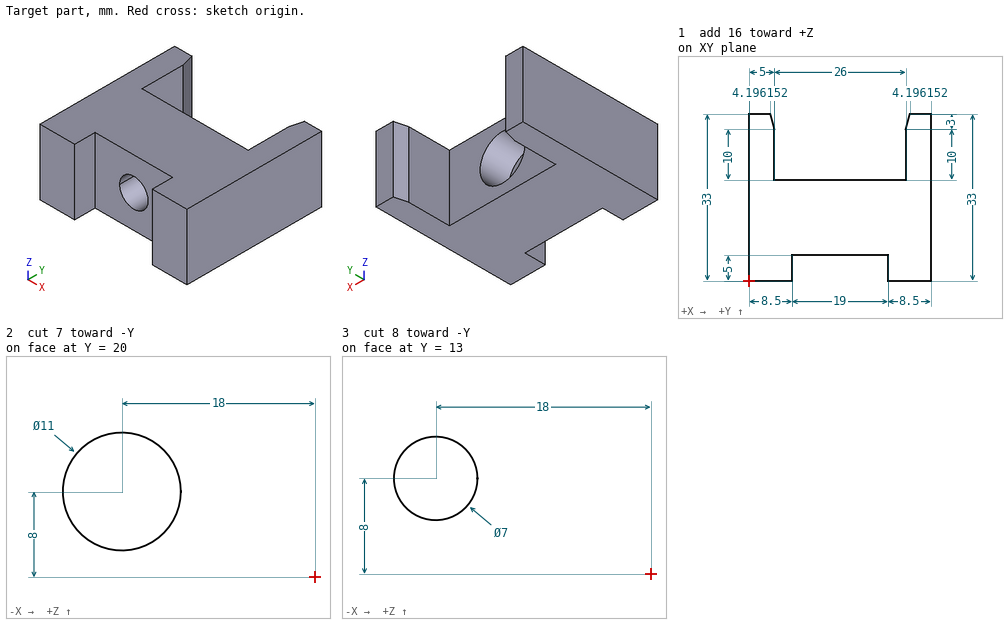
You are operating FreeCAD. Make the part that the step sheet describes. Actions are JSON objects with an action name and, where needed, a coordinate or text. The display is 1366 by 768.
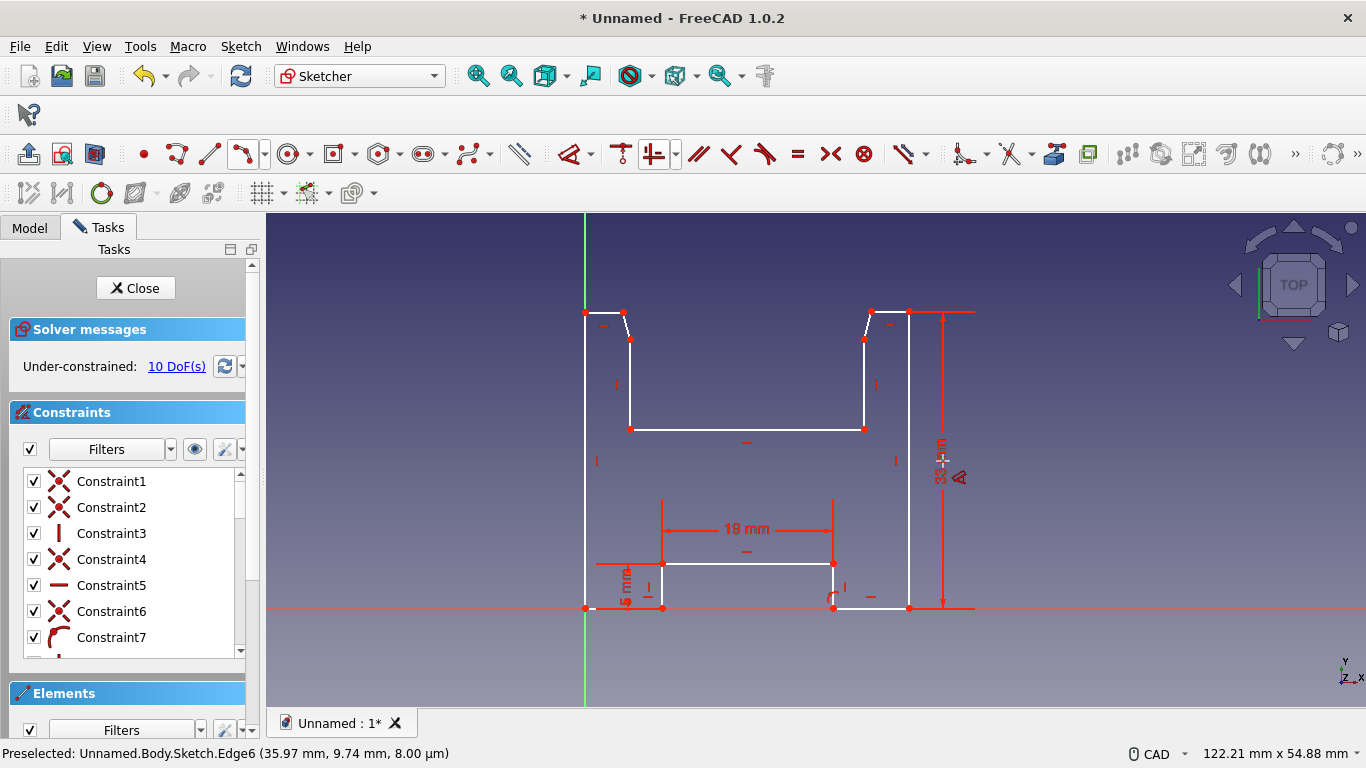
{"action": "left_click", "coordinate": [864, 367]}
{"action": "left_click", "coordinate": [830, 385]}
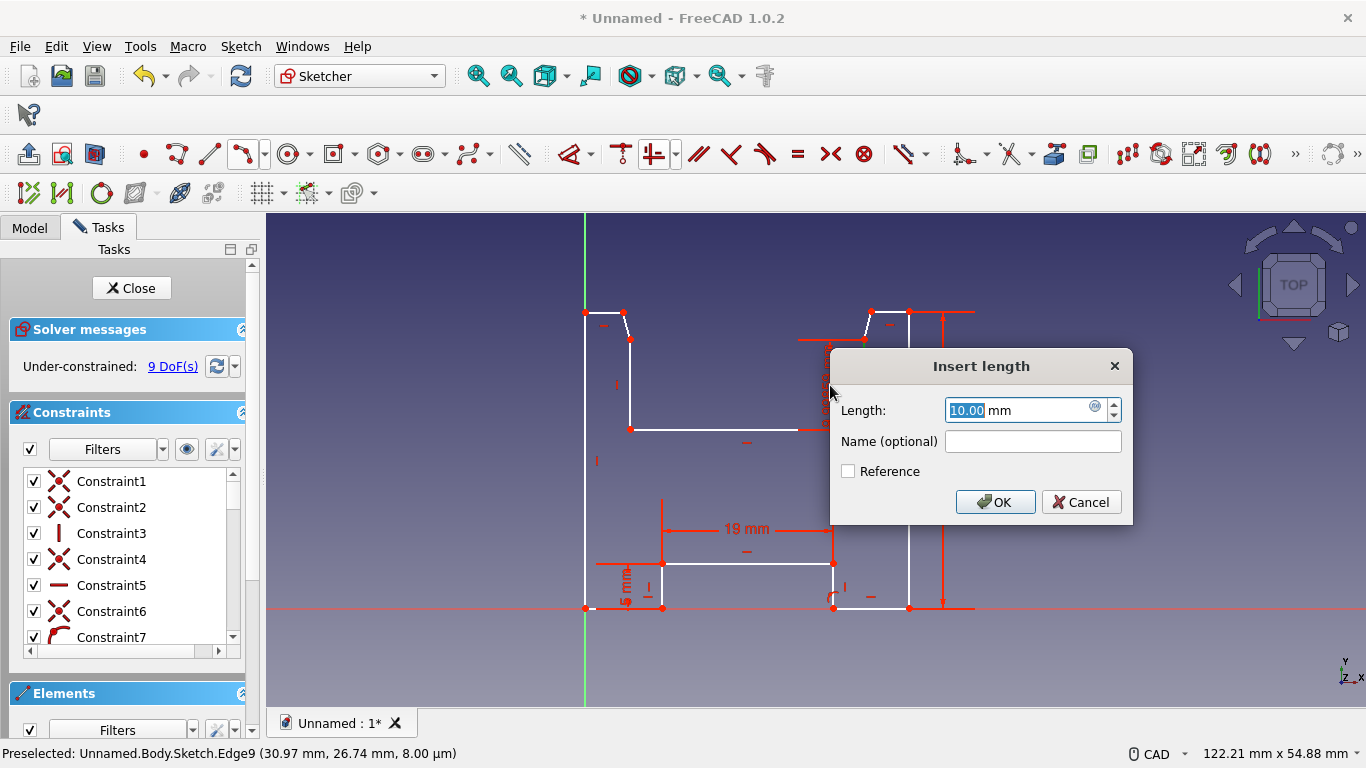
{"action": "type", "text": "10"}
{"action": "key", "text": "Return"}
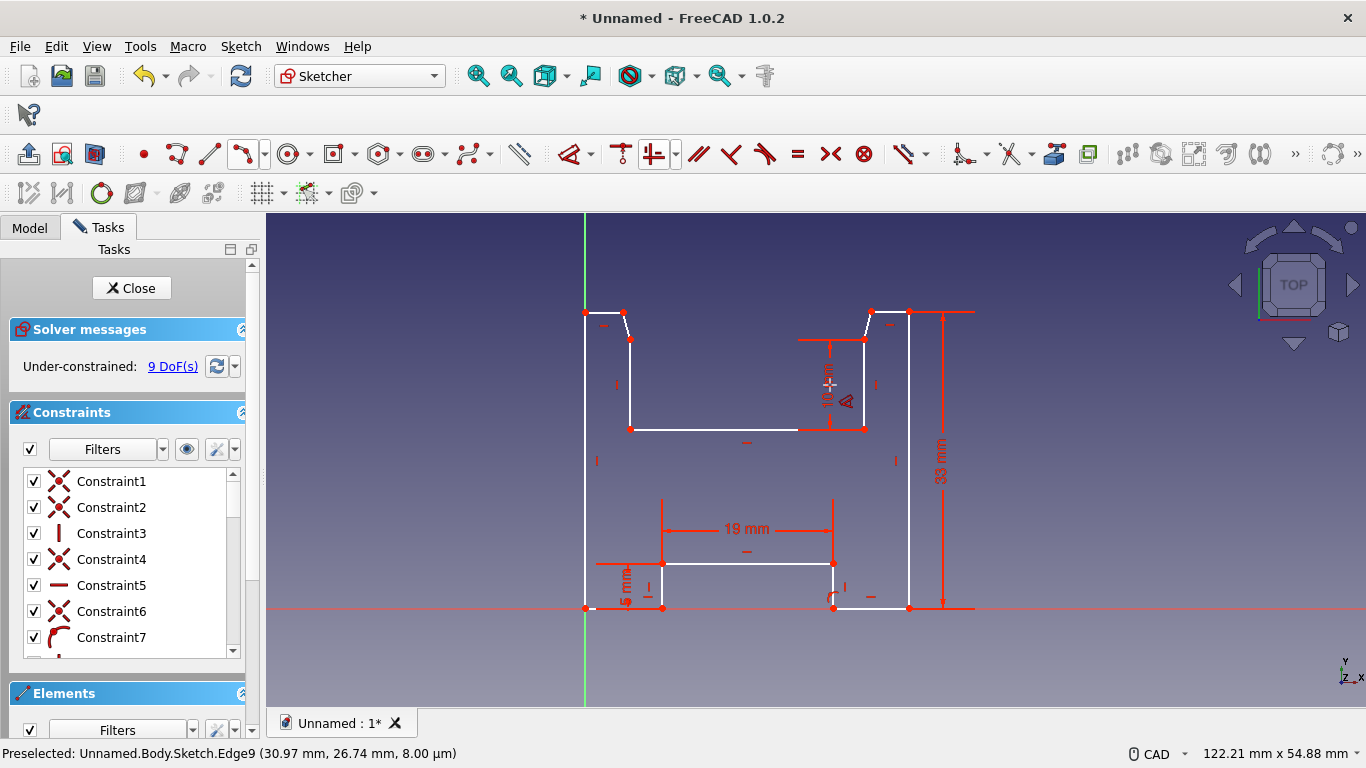
{"action": "left_click", "coordinate": [794, 430]}
{"action": "left_click", "coordinate": [747, 396]}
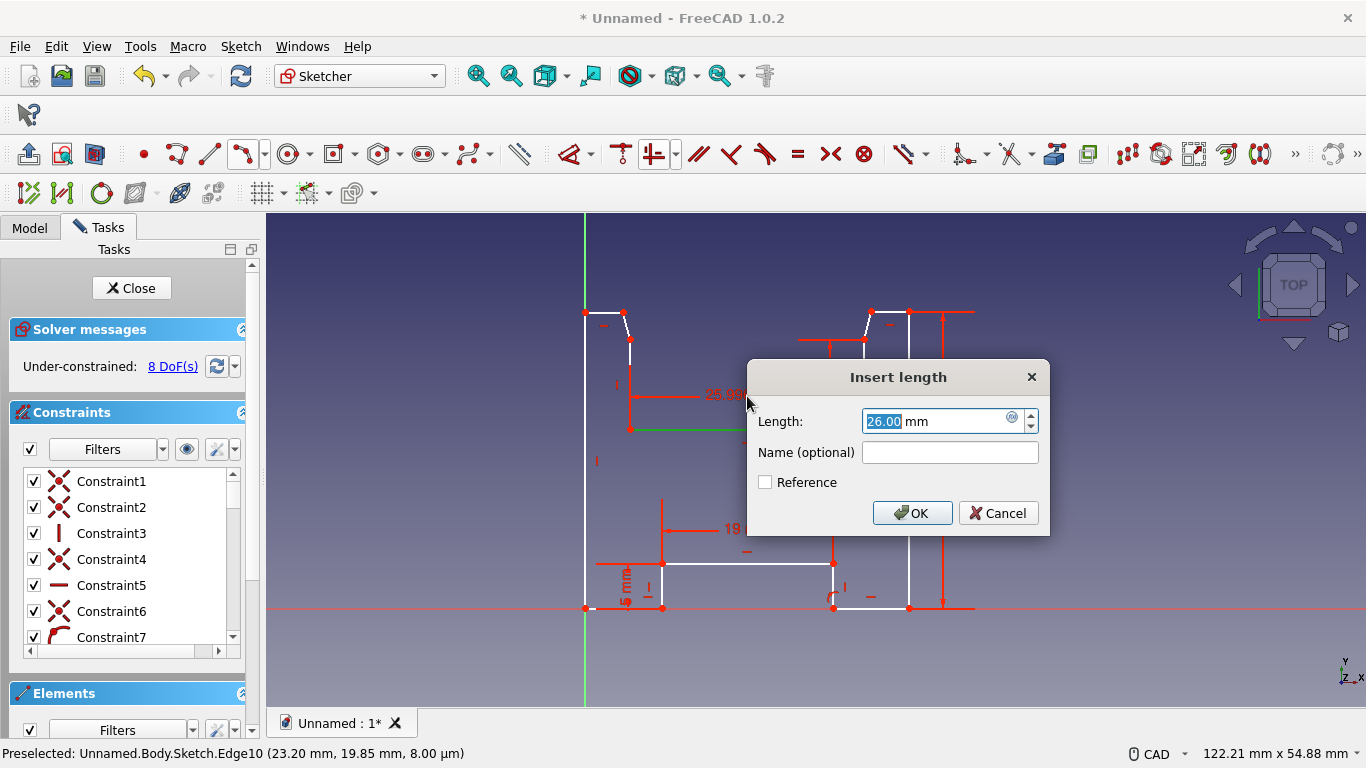
{"action": "type", "text": "26"}
{"action": "key", "text": "Return"}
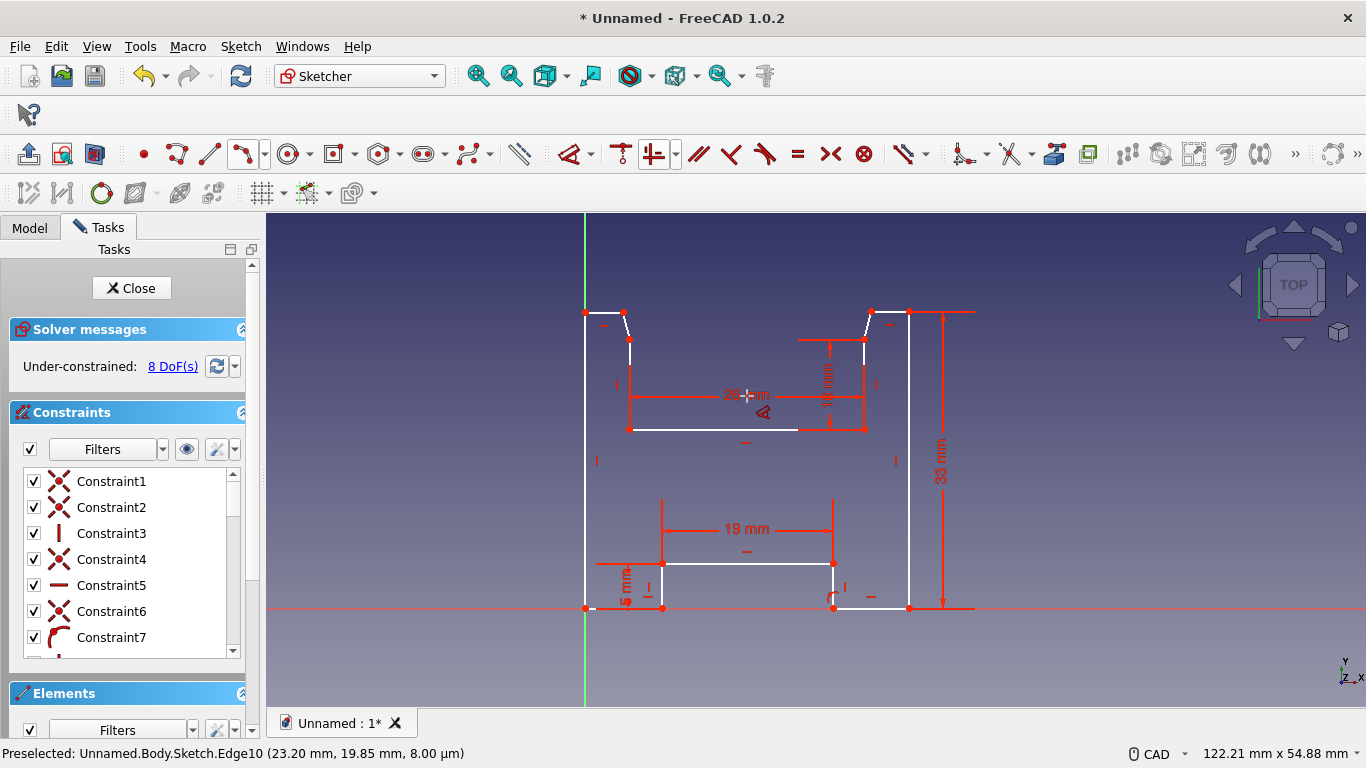
{"action": "left_click", "coordinate": [630, 403]}
{"action": "left_click", "coordinate": [664, 385]}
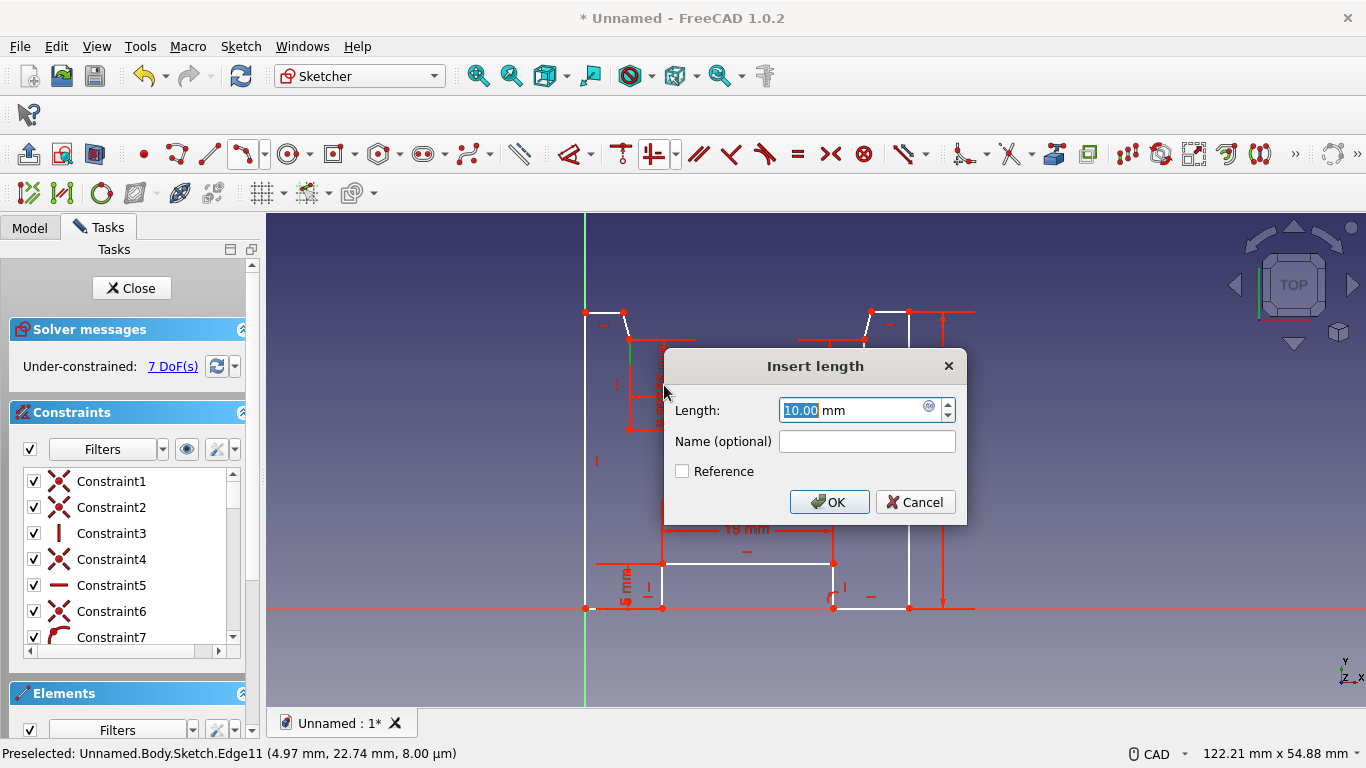
{"action": "type", "text": "10"}
{"action": "key", "text": "Return"}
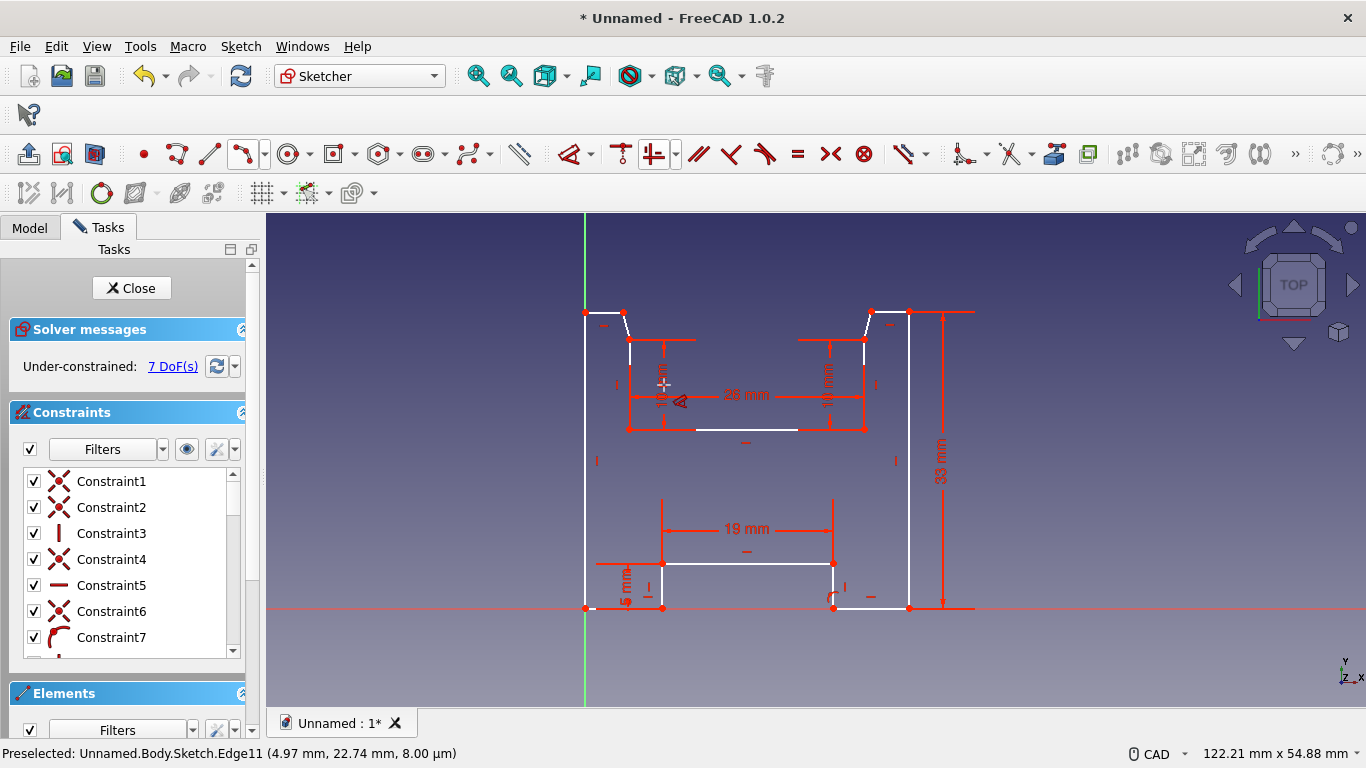
{"action": "left_click", "coordinate": [585, 402]}
{"action": "left_click", "coordinate": [551, 461]}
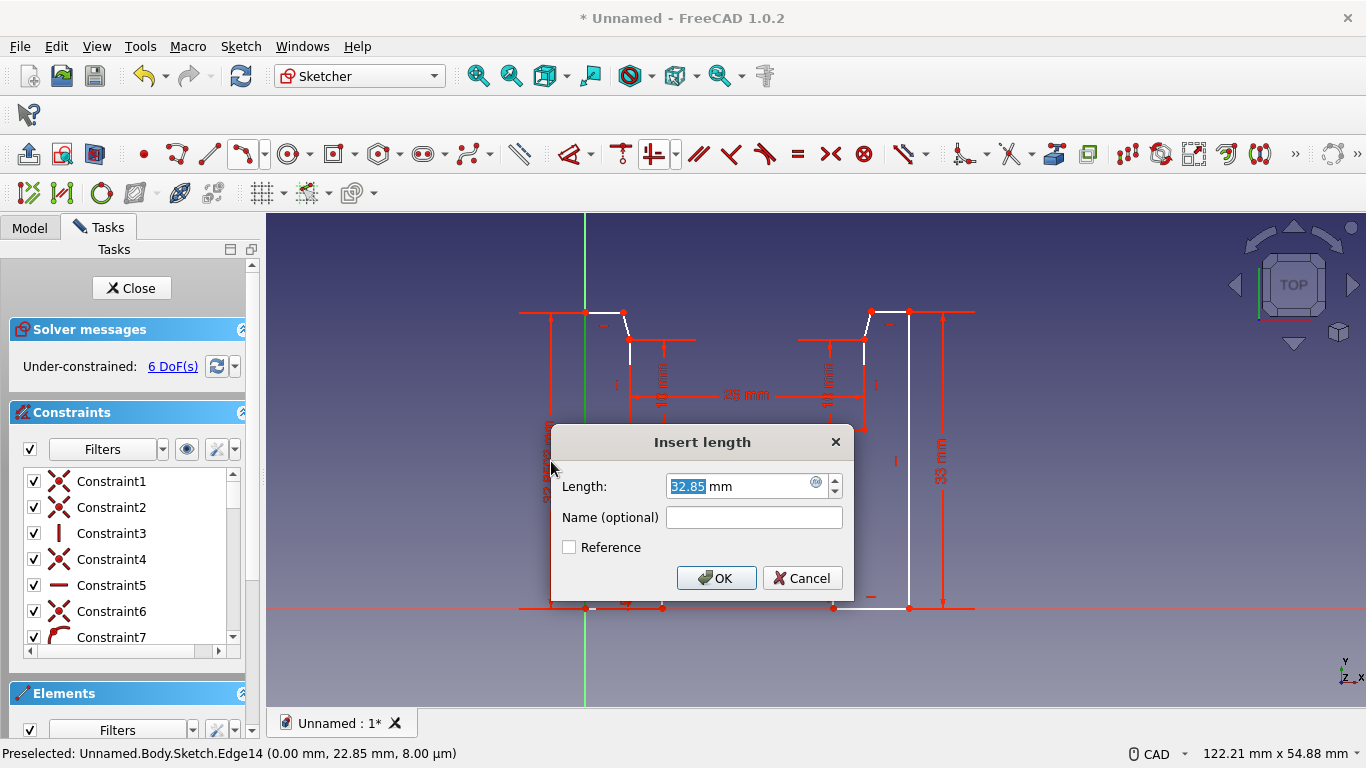
{"action": "type", "text": "33"}
{"action": "key", "text": "Return"}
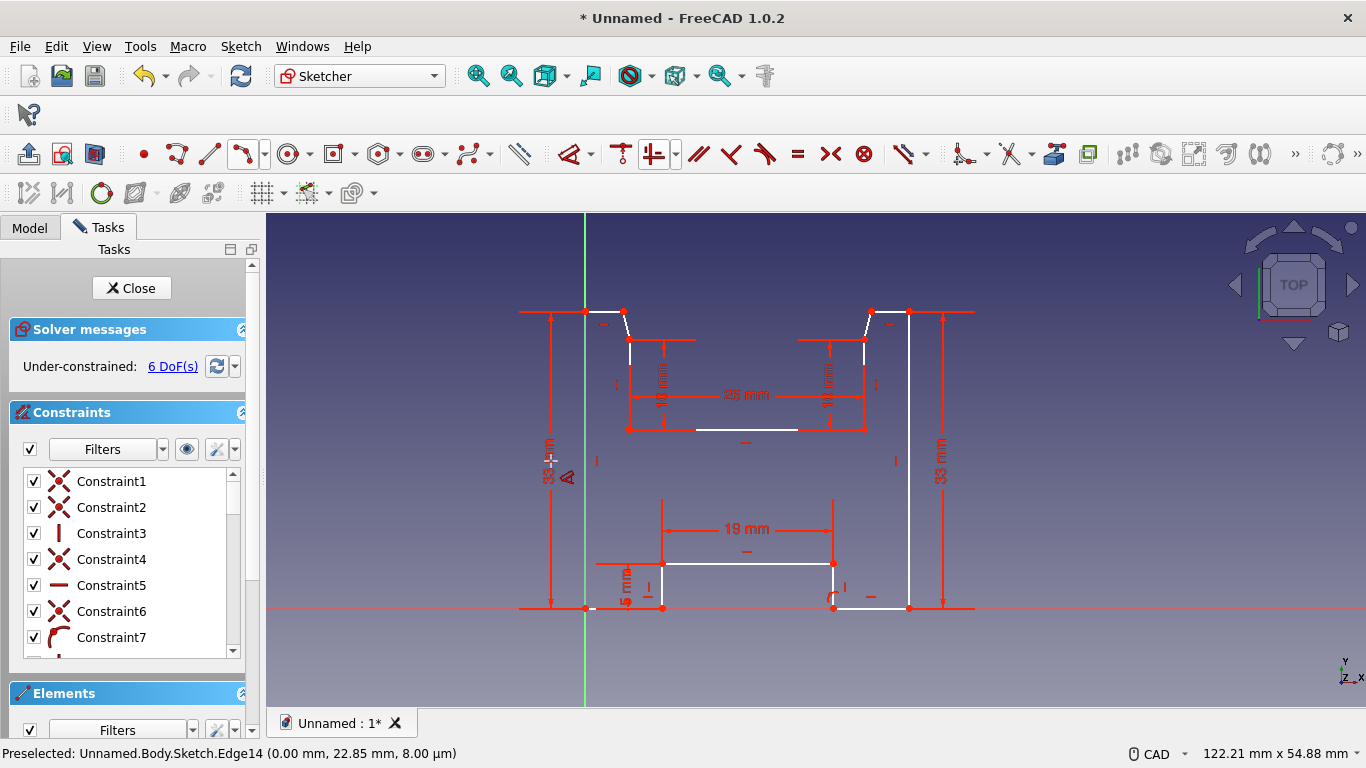
{"action": "left_click", "coordinate": [630, 430]}
{"action": "left_click", "coordinate": [608, 643]}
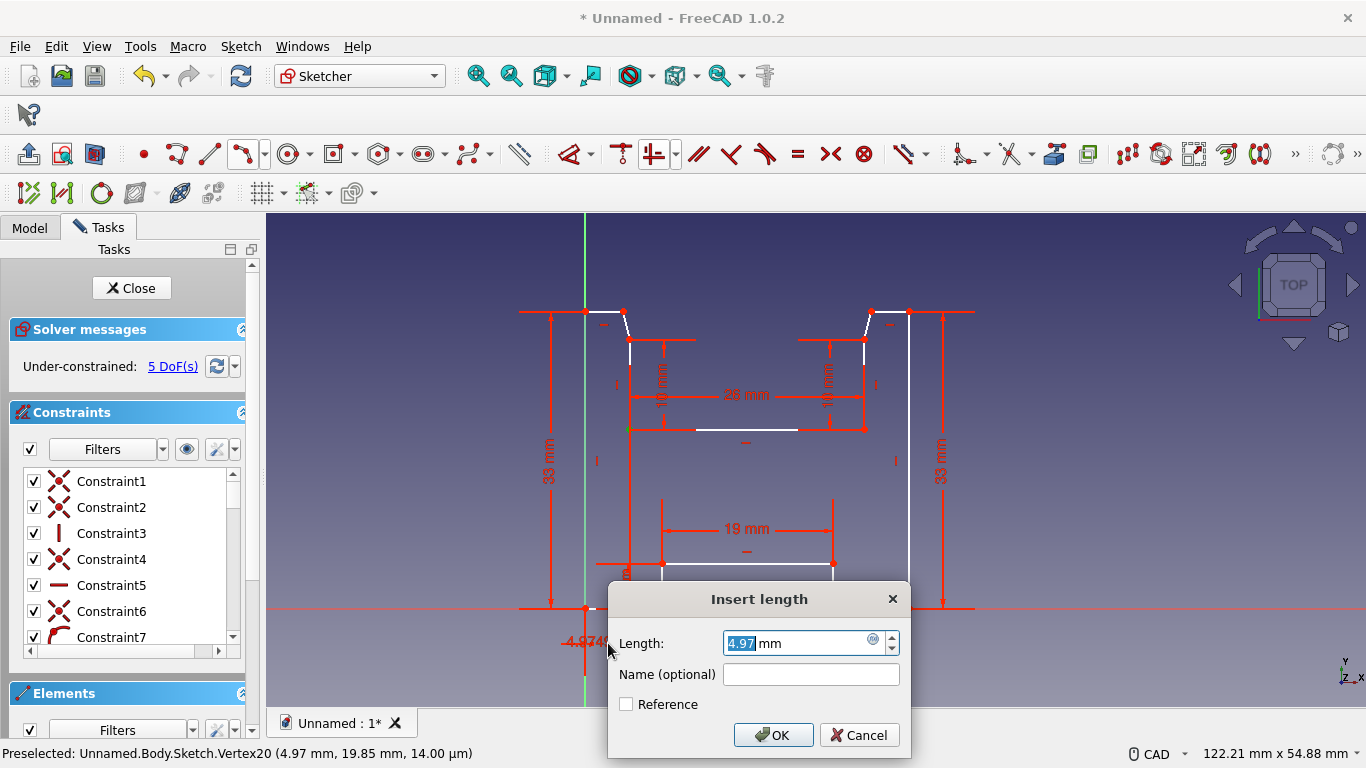
{"action": "type", "text": "5"}
{"action": "key", "text": "Return"}